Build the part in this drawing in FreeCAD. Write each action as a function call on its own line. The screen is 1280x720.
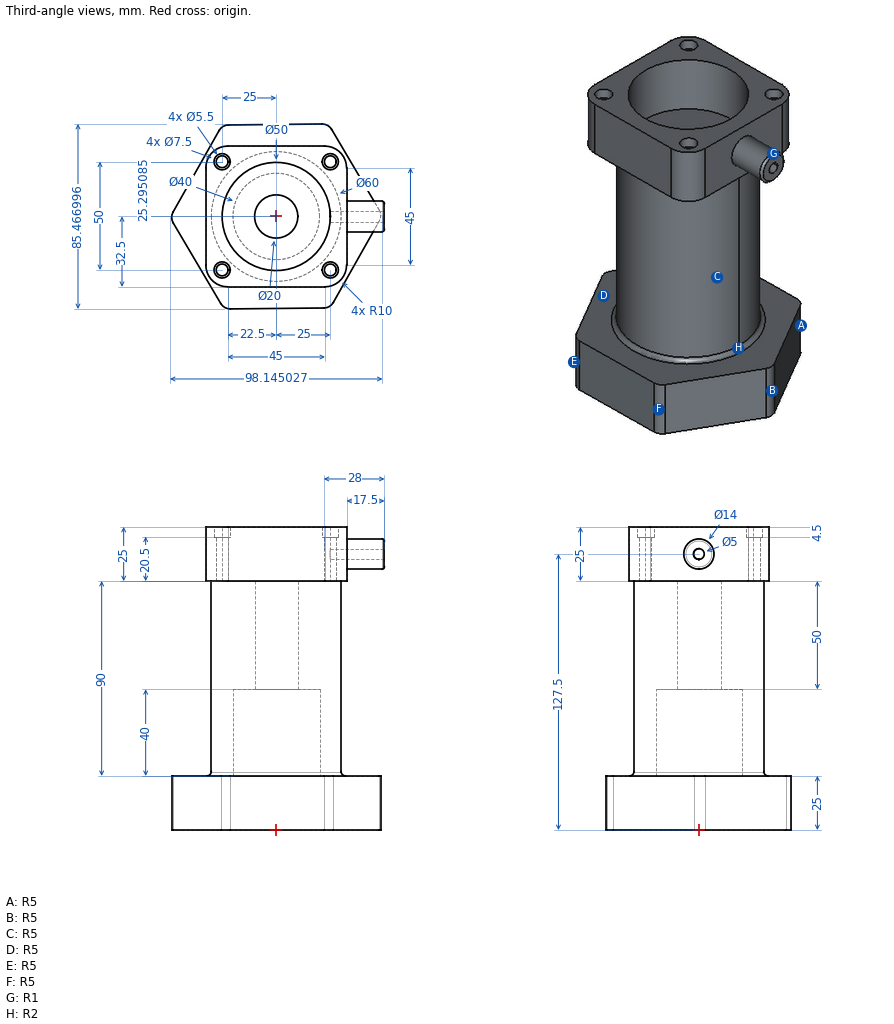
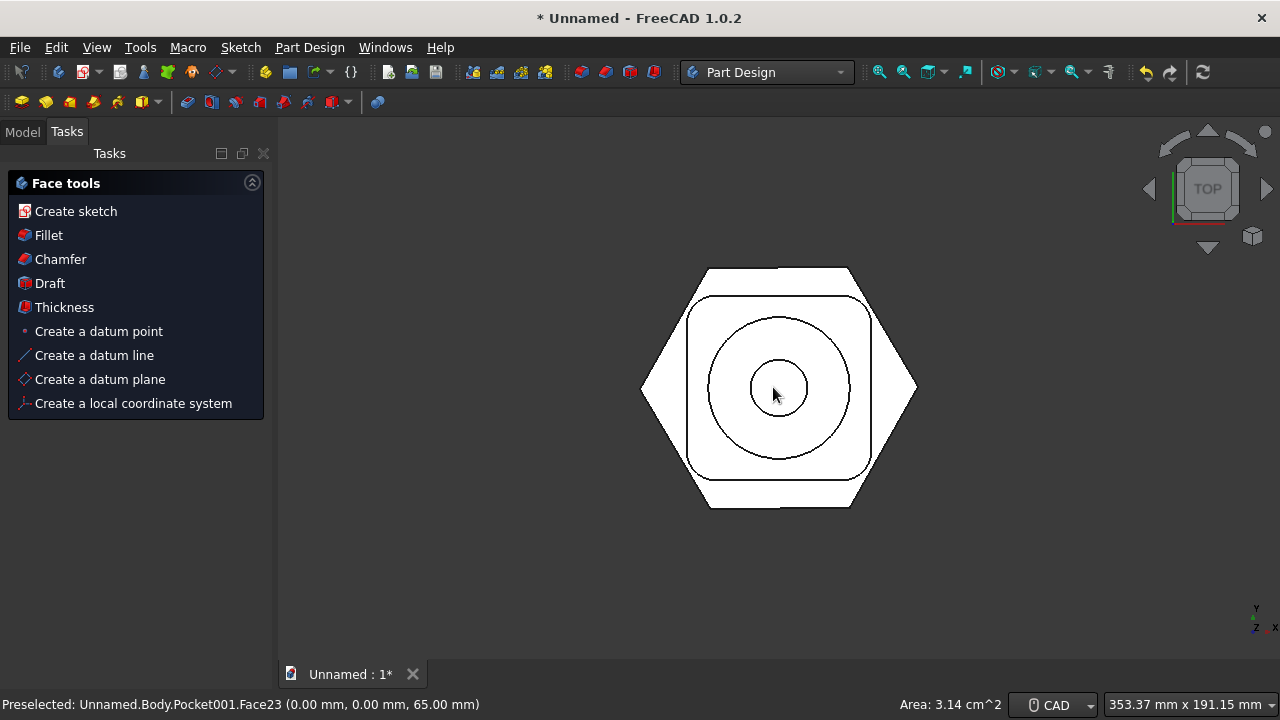
click(84, 72)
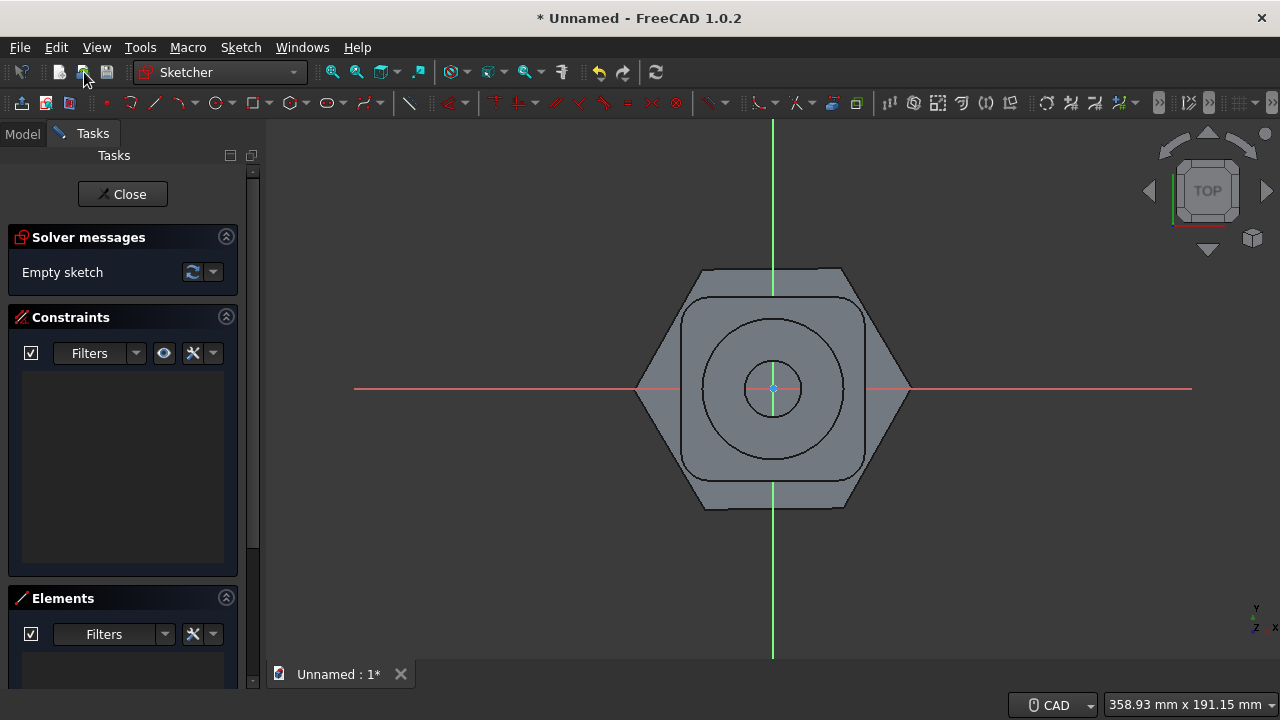
key(q)
key(s)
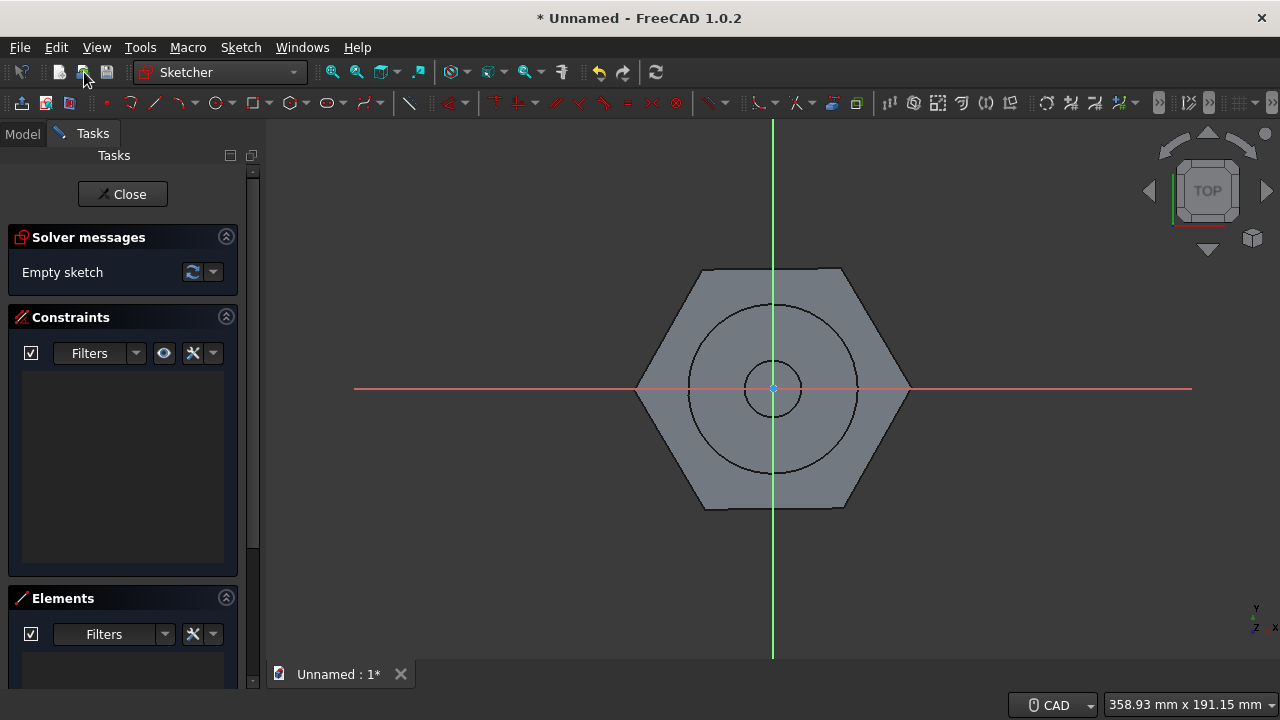
scroll(803, 389, up, 6)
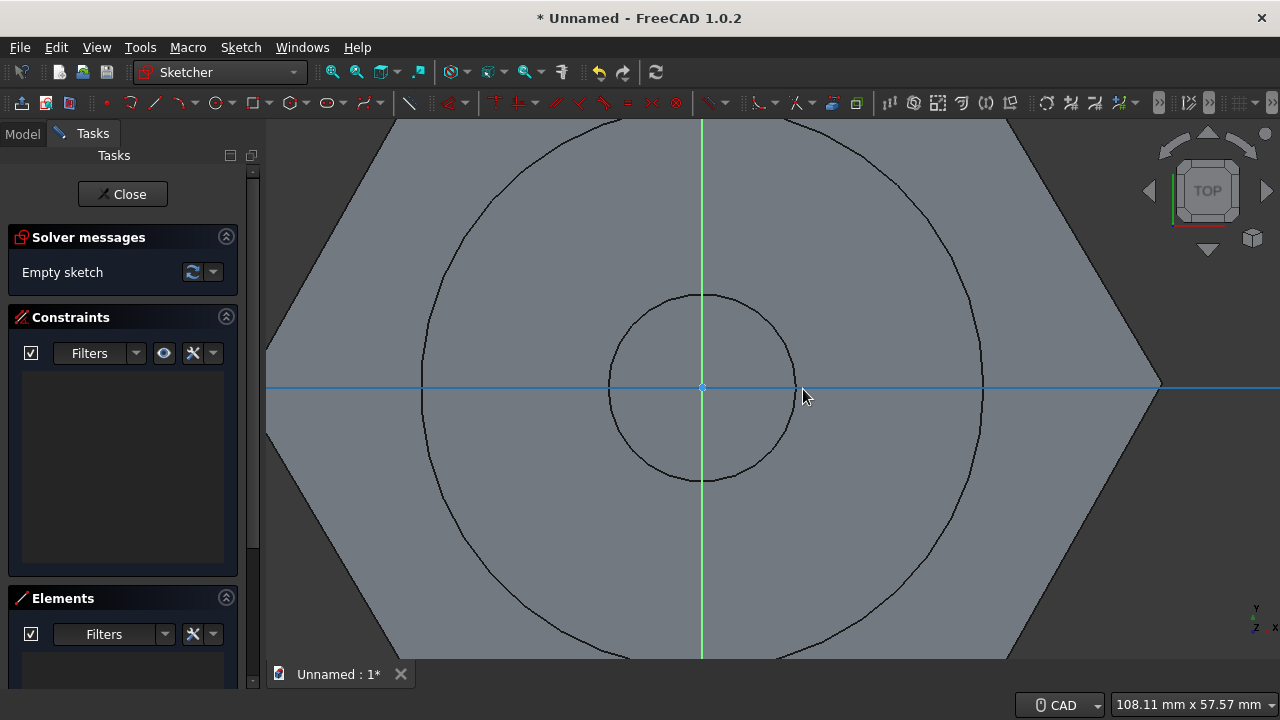
click(216, 104)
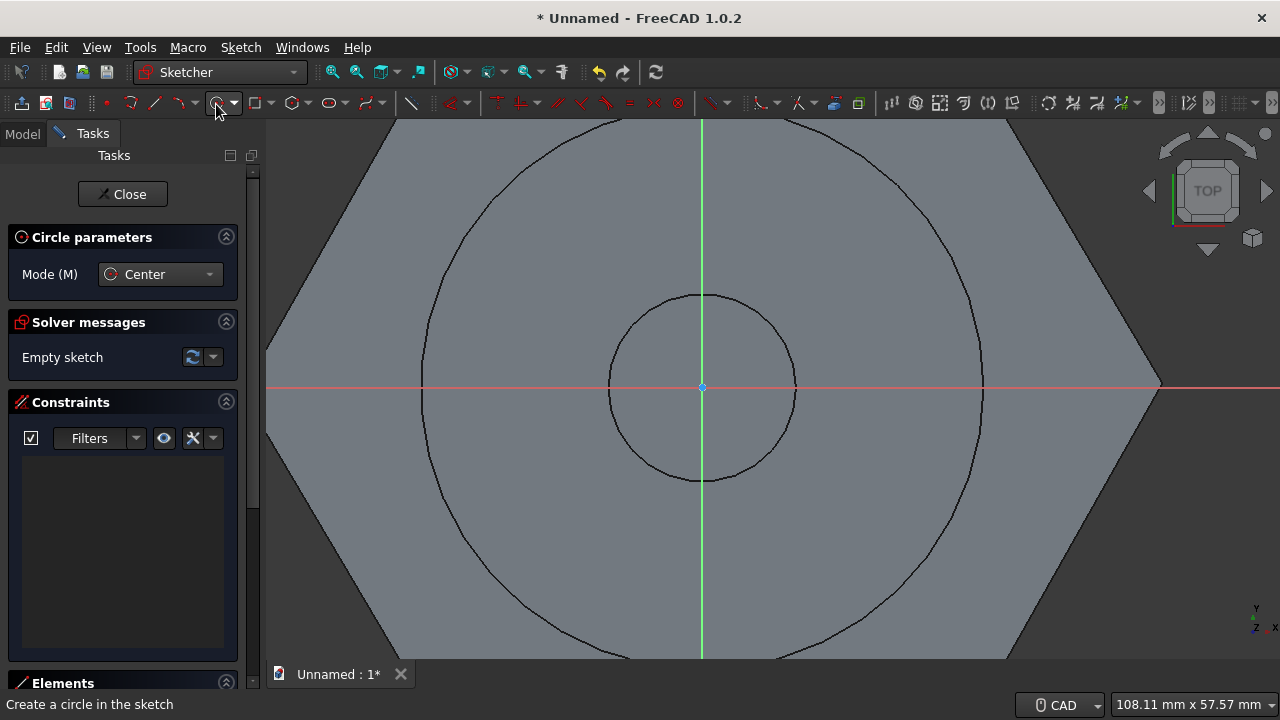
click(702, 388)
click(835, 255)
key(Escape)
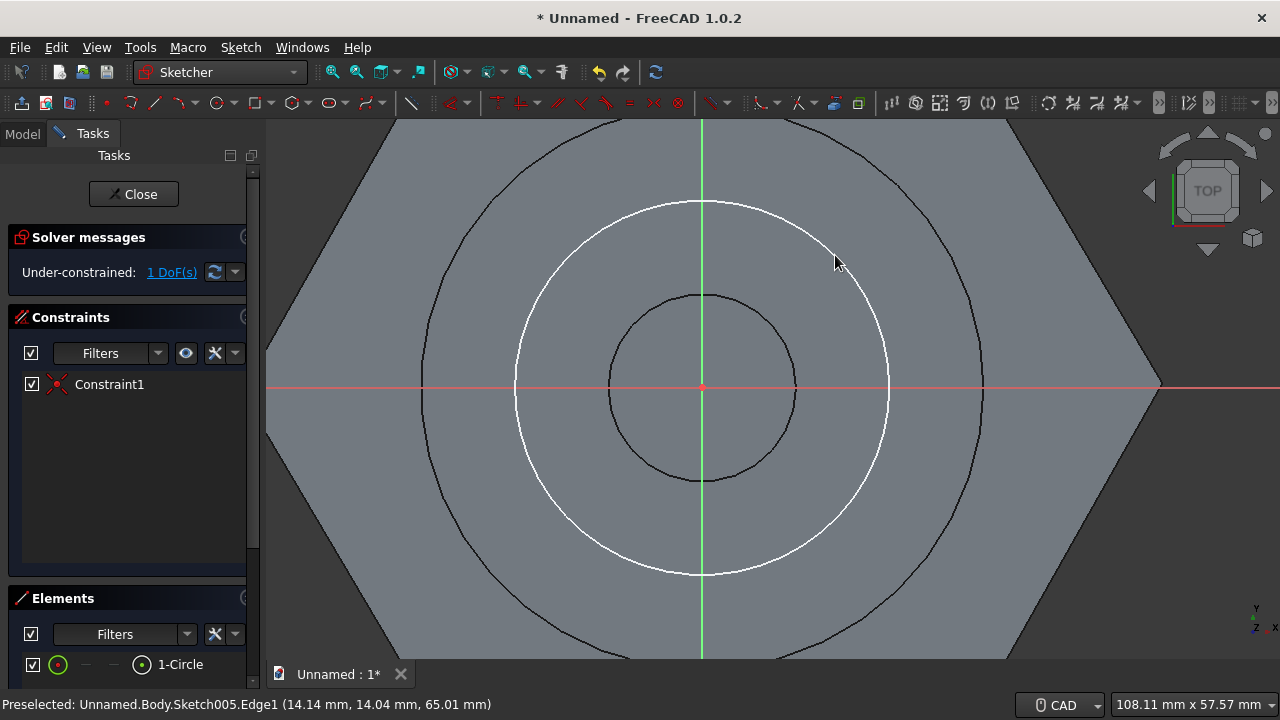
click(450, 104)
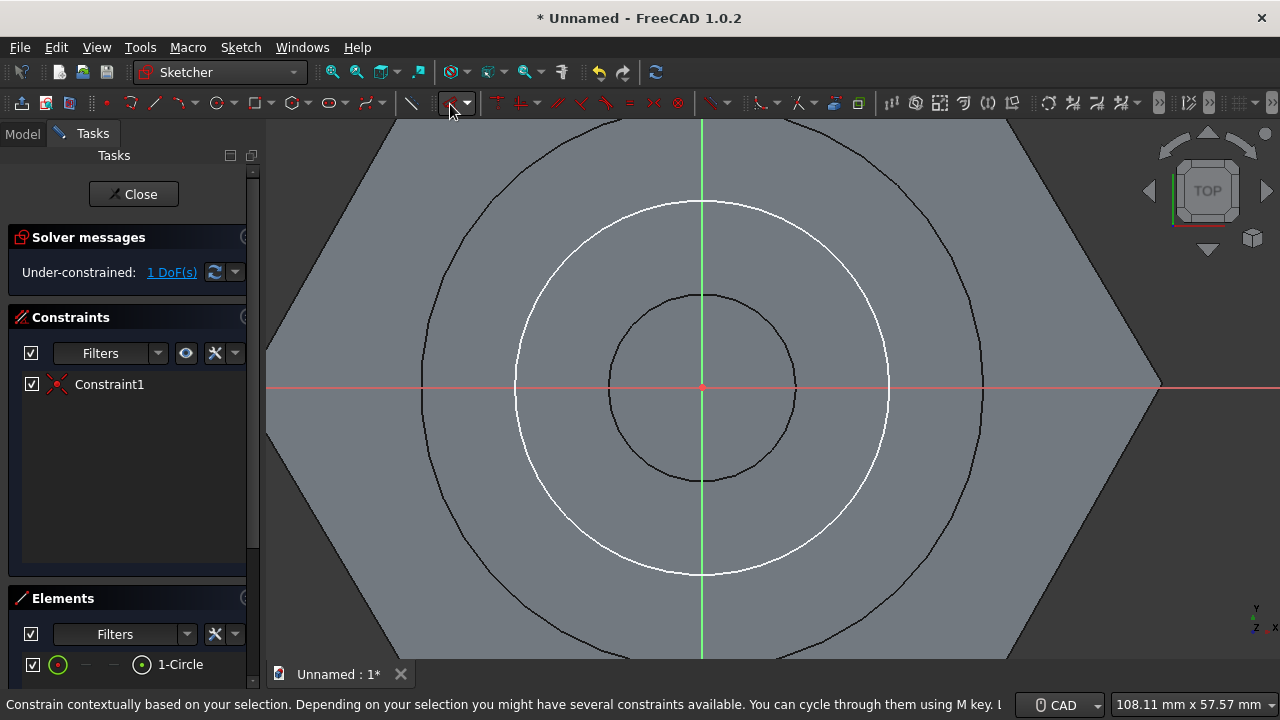
click(834, 255)
click(857, 232)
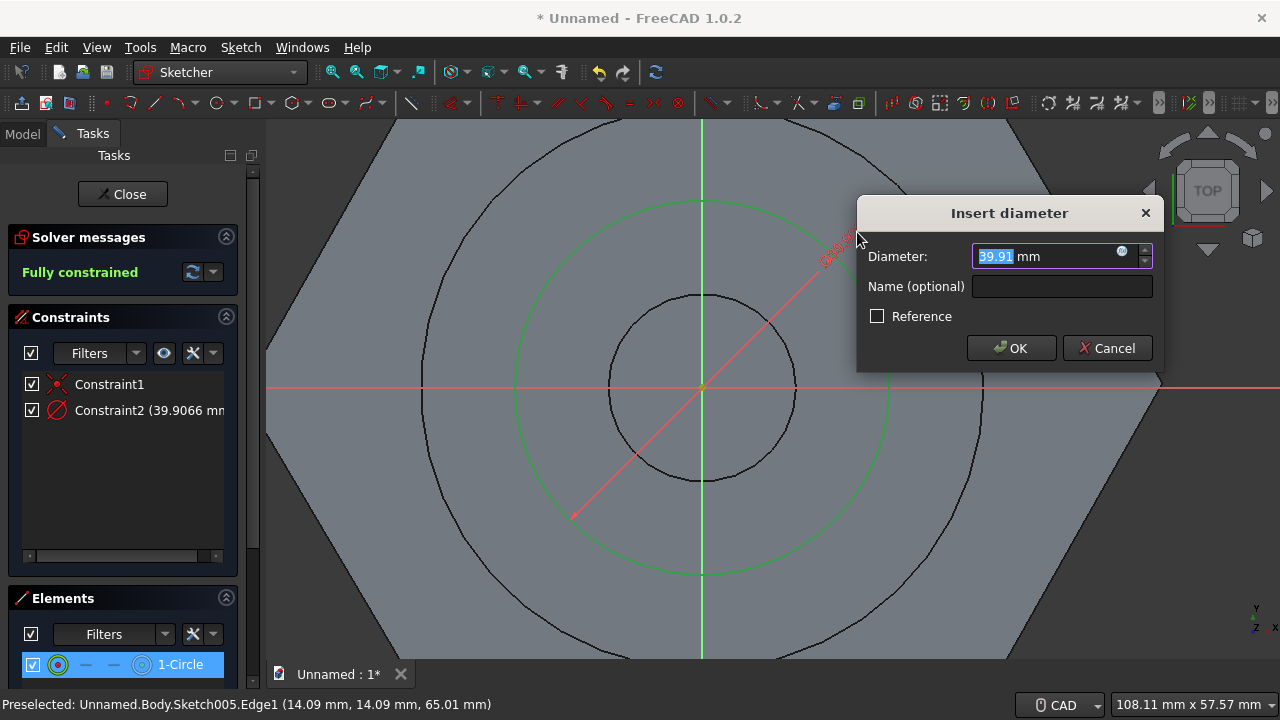
text(40)
key(Return)
key(Escape)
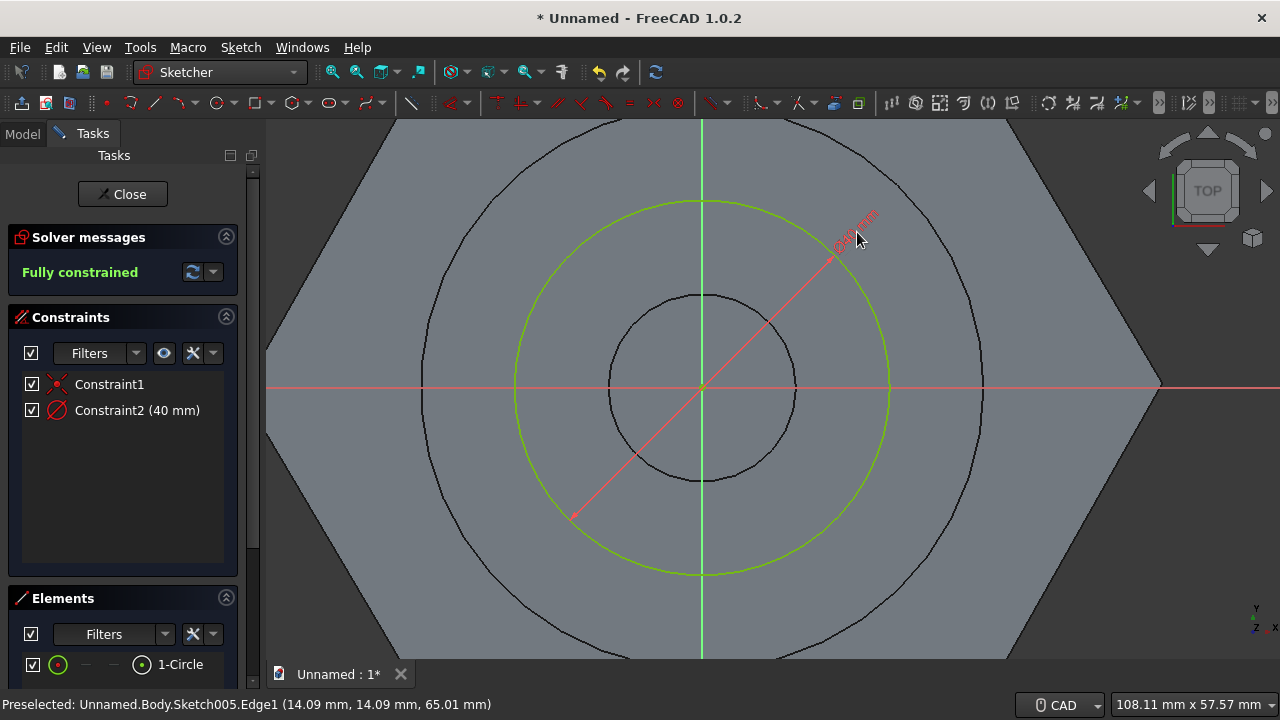
click(123, 194)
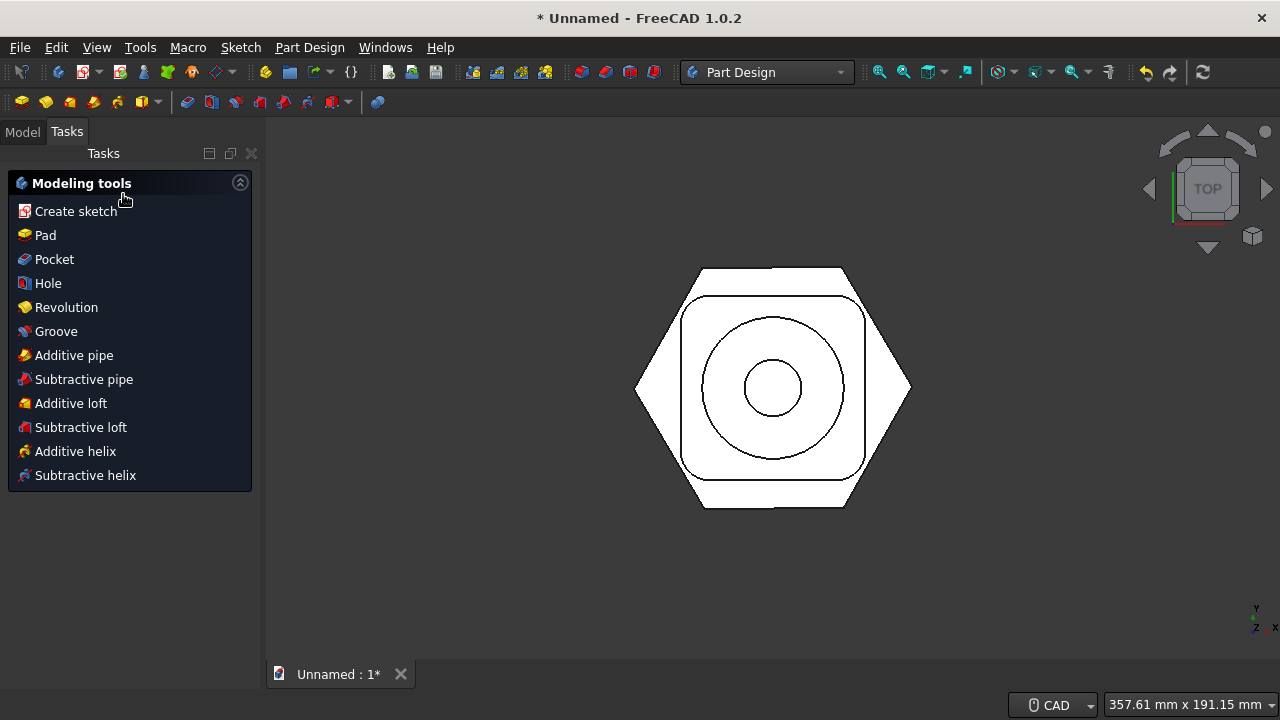
click(188, 102)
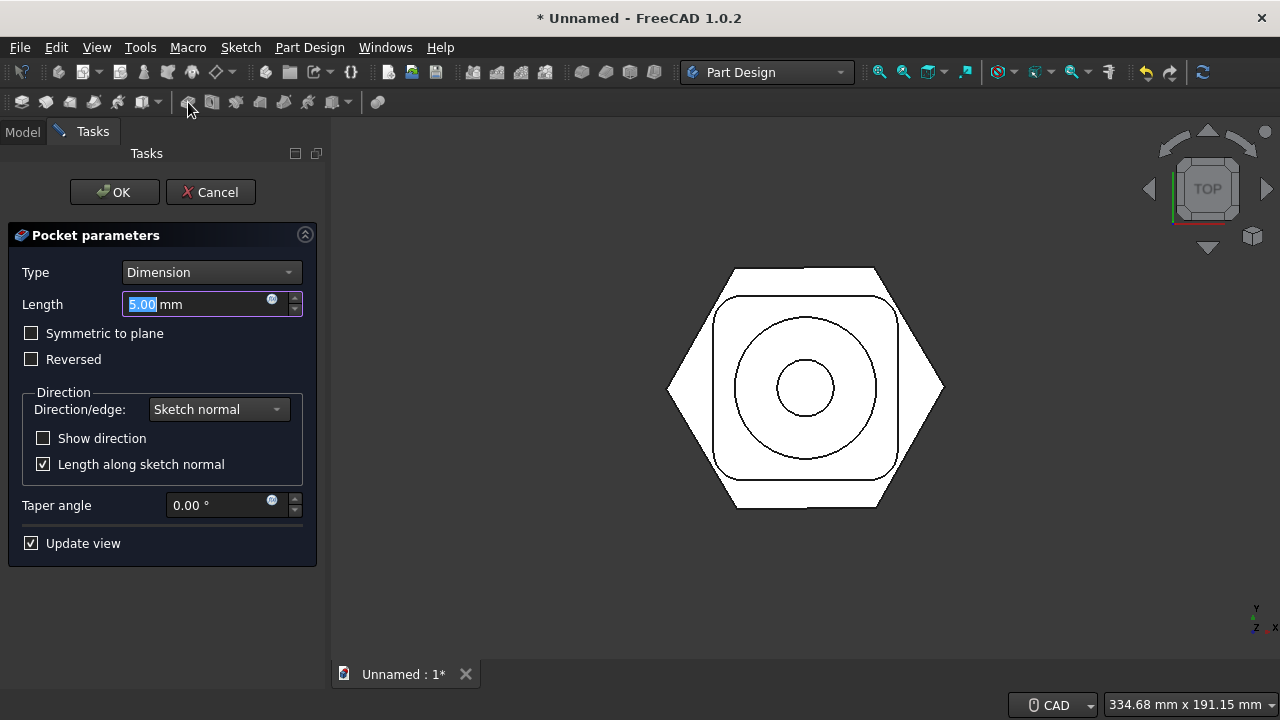
text(40)
key(Tab)